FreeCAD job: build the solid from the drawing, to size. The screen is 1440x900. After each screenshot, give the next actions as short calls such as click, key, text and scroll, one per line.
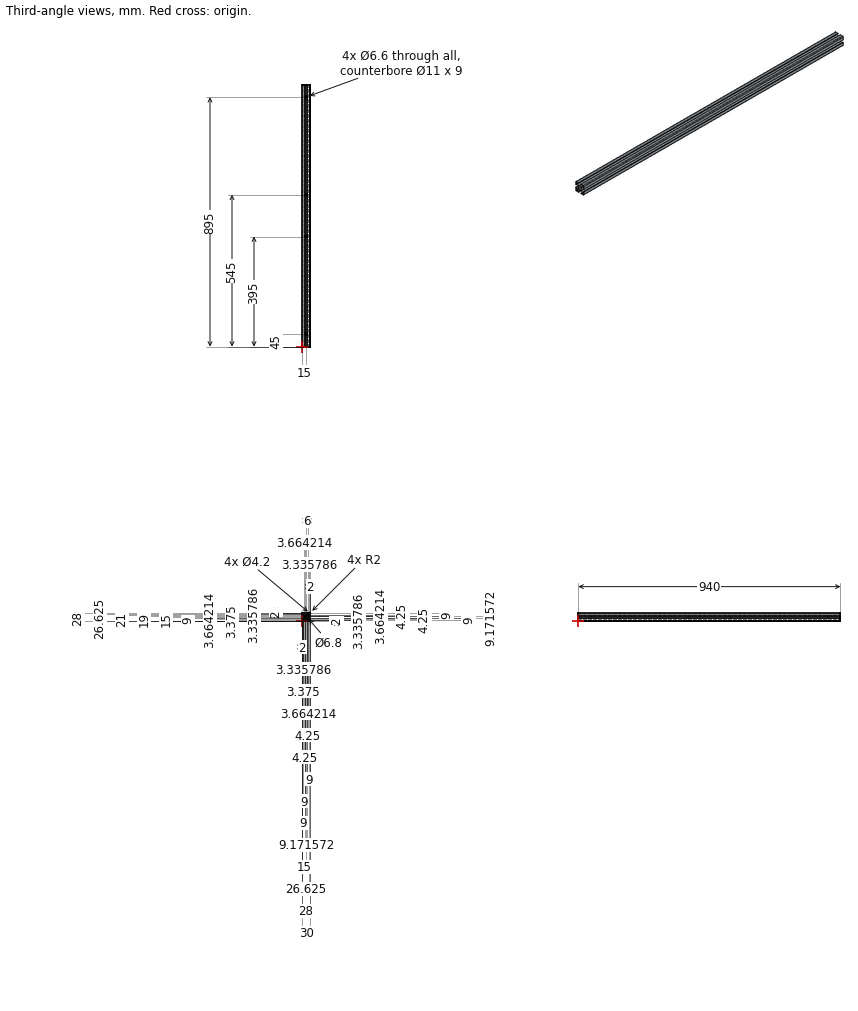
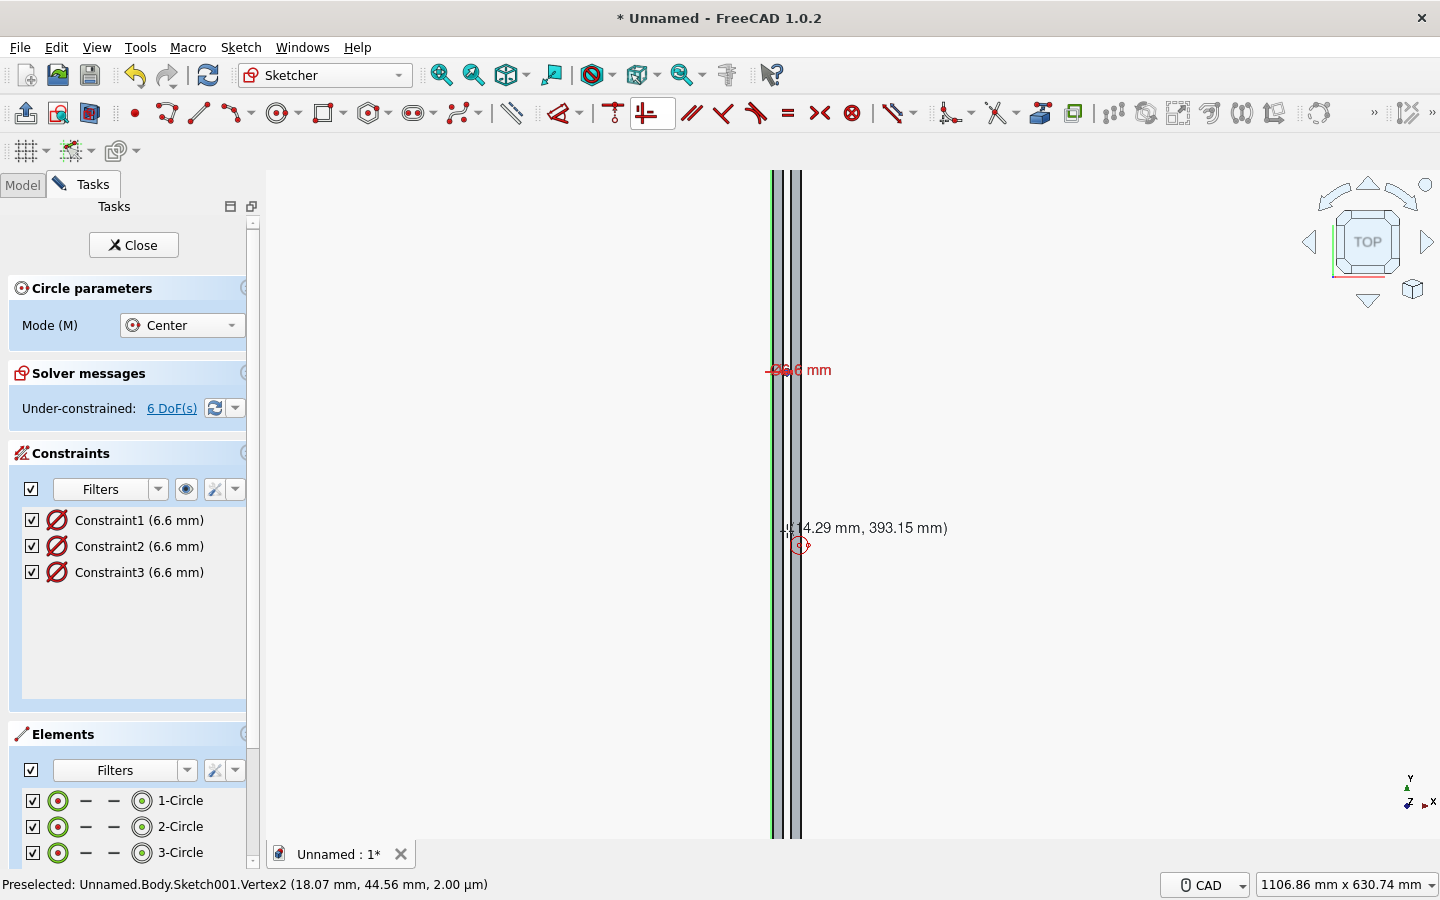
click(787, 531)
move(790, 528)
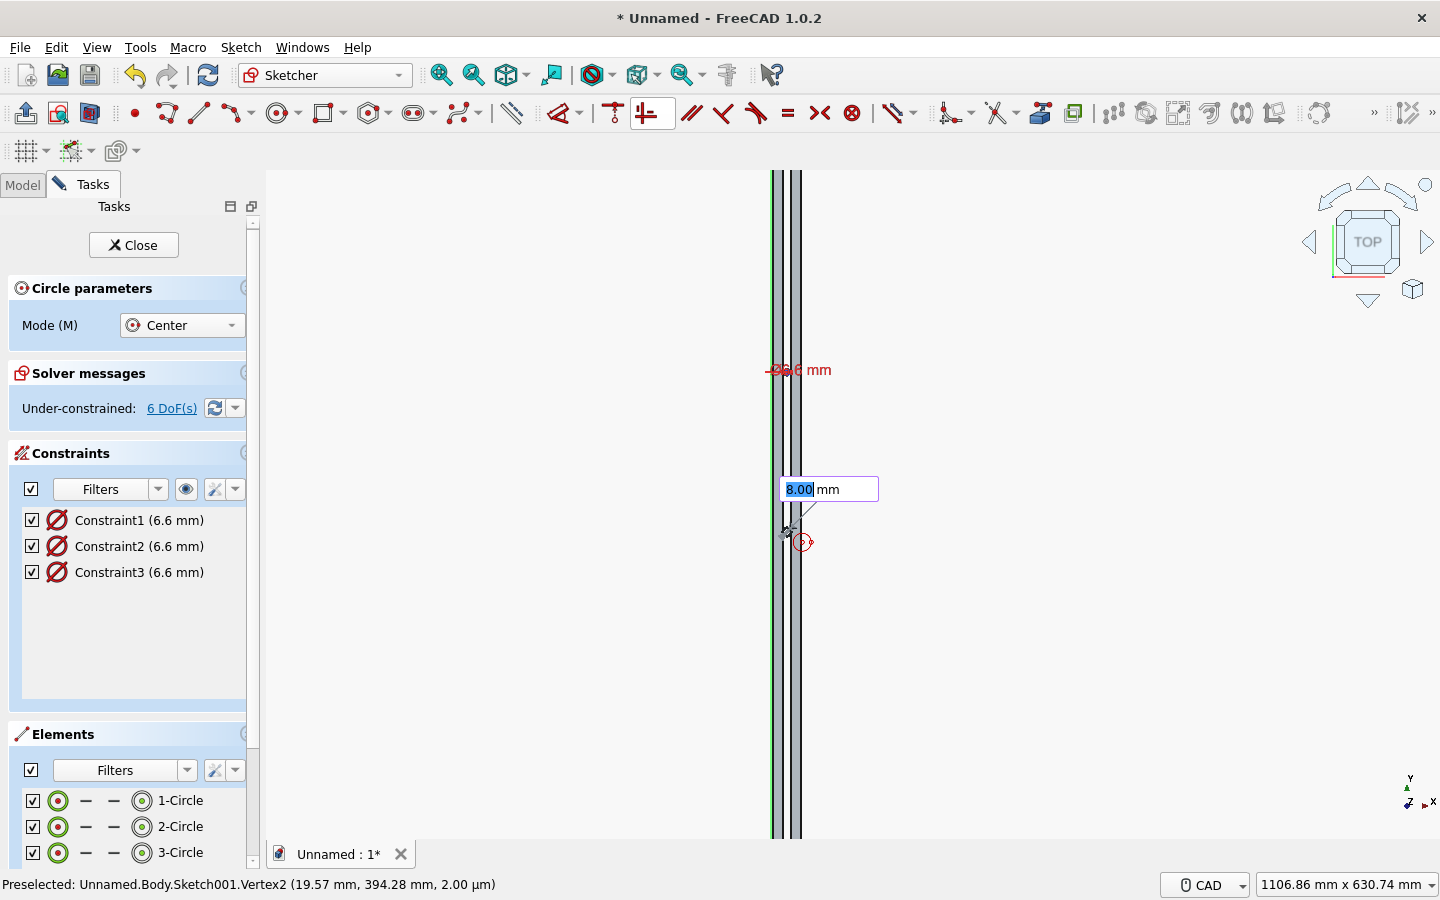
text(6.6)
key(Return)
key(Escape)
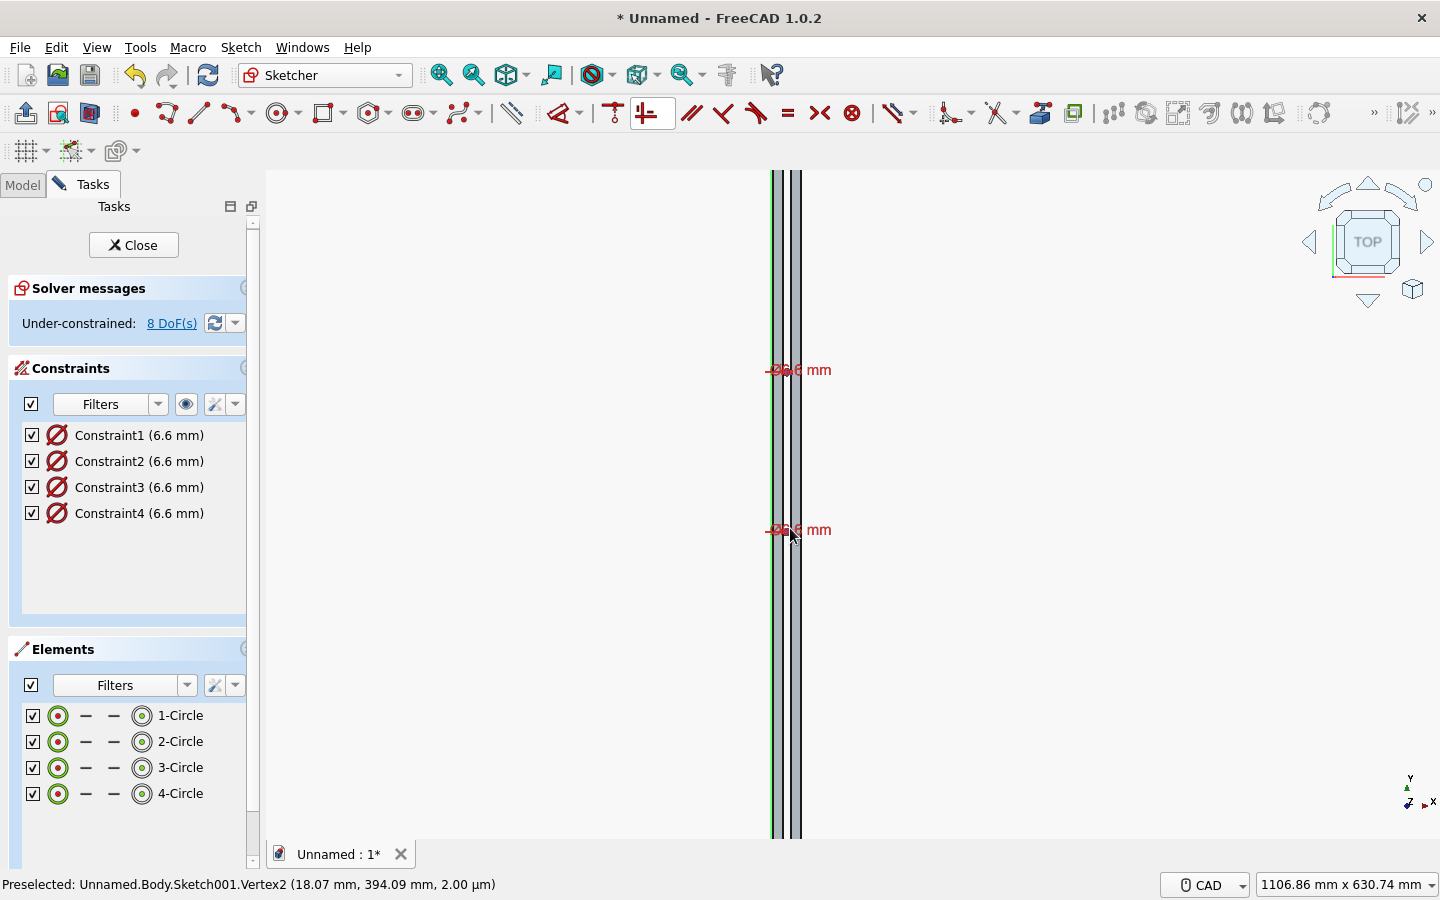
click(558, 114)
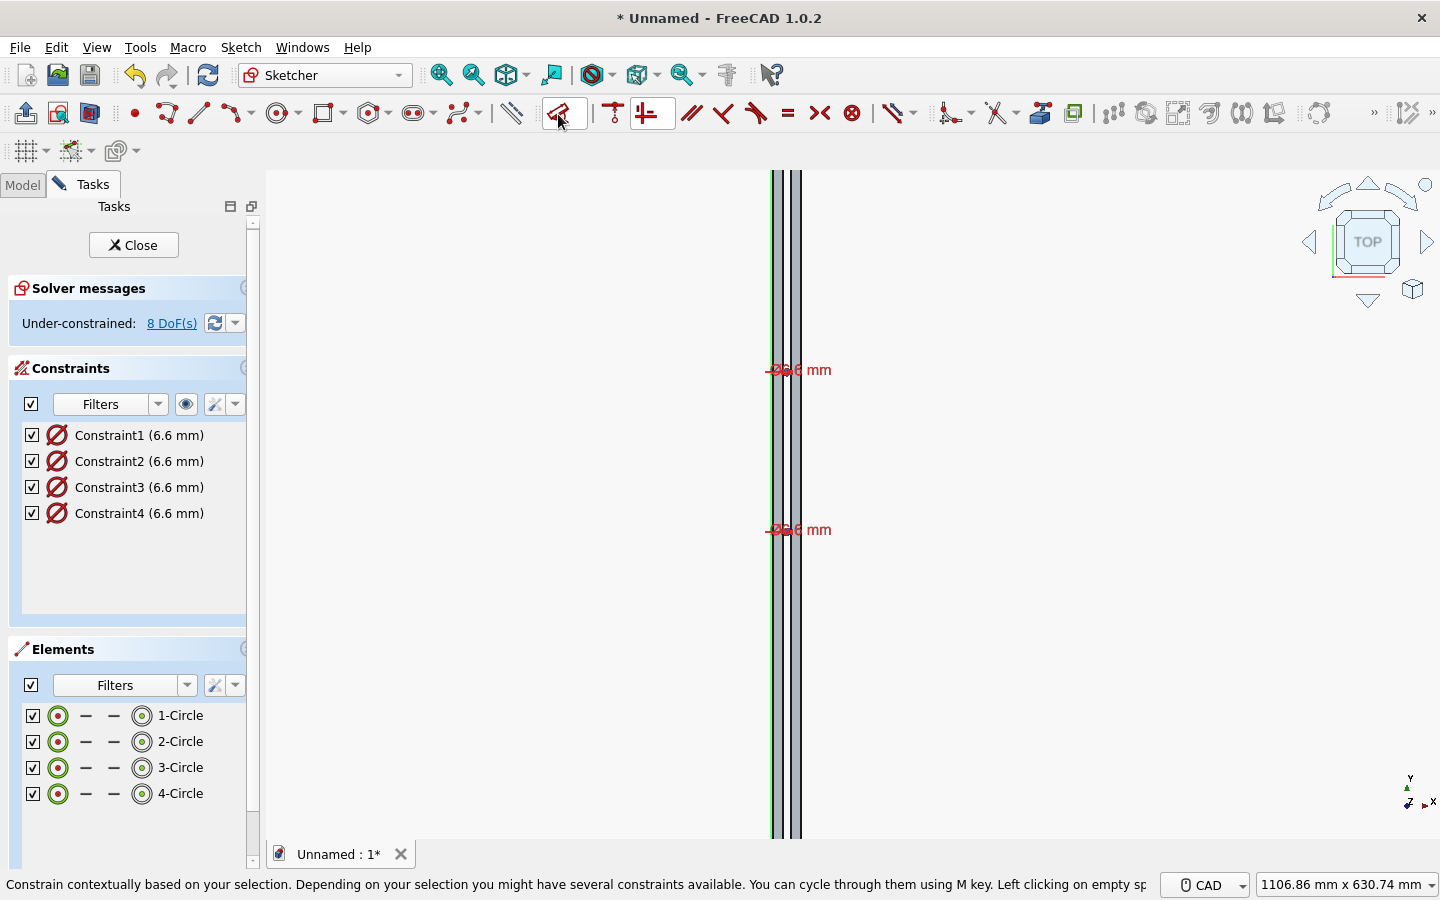
scroll(787, 530, down, 4)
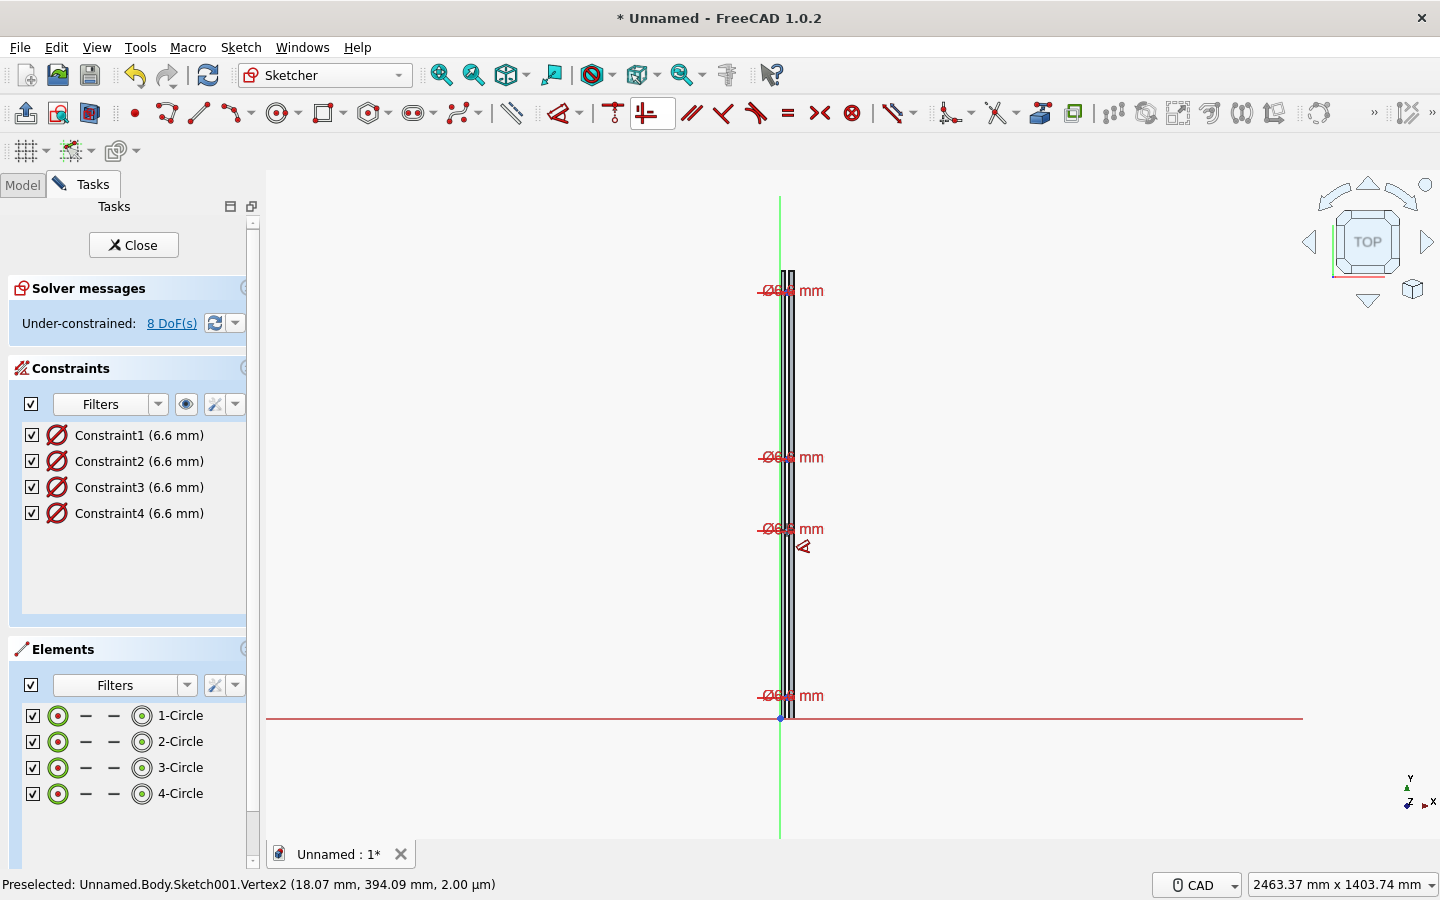
scroll(787, 293, up, 9)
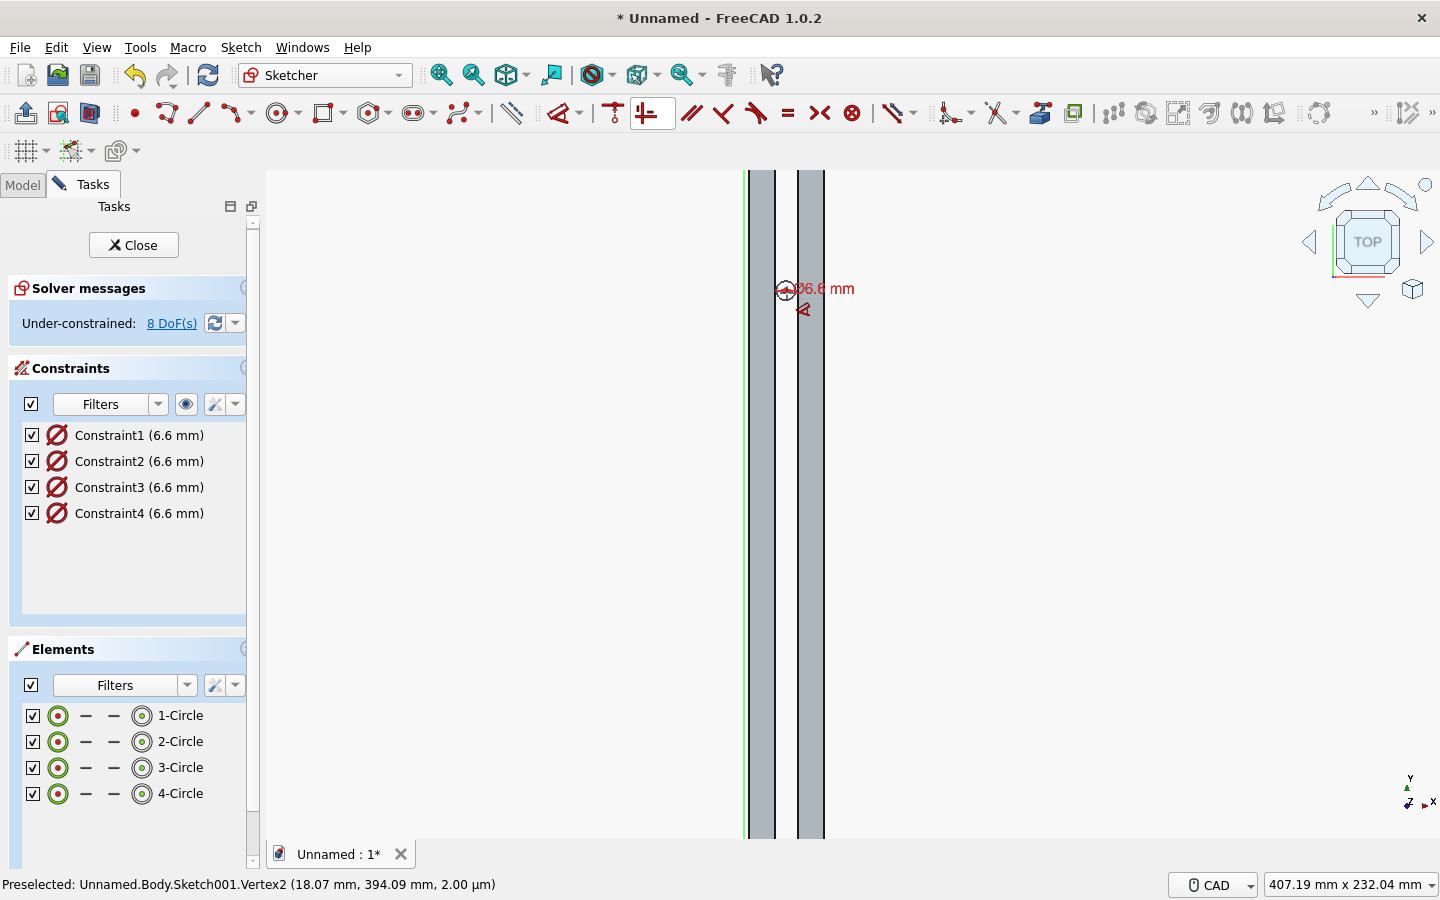
click(786, 291)
click(765, 257)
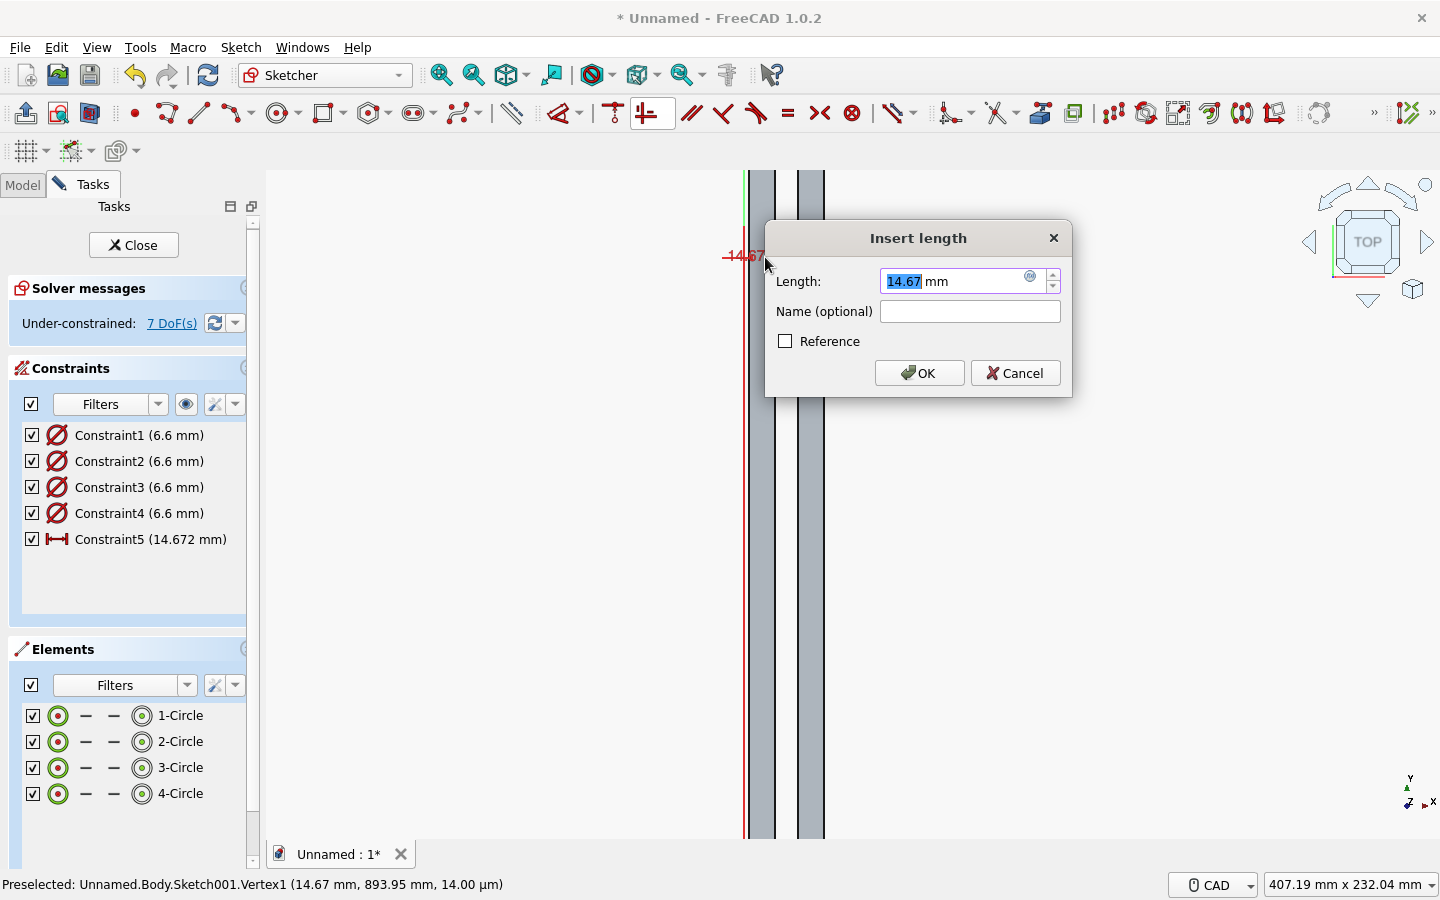
text(15)
key(Return)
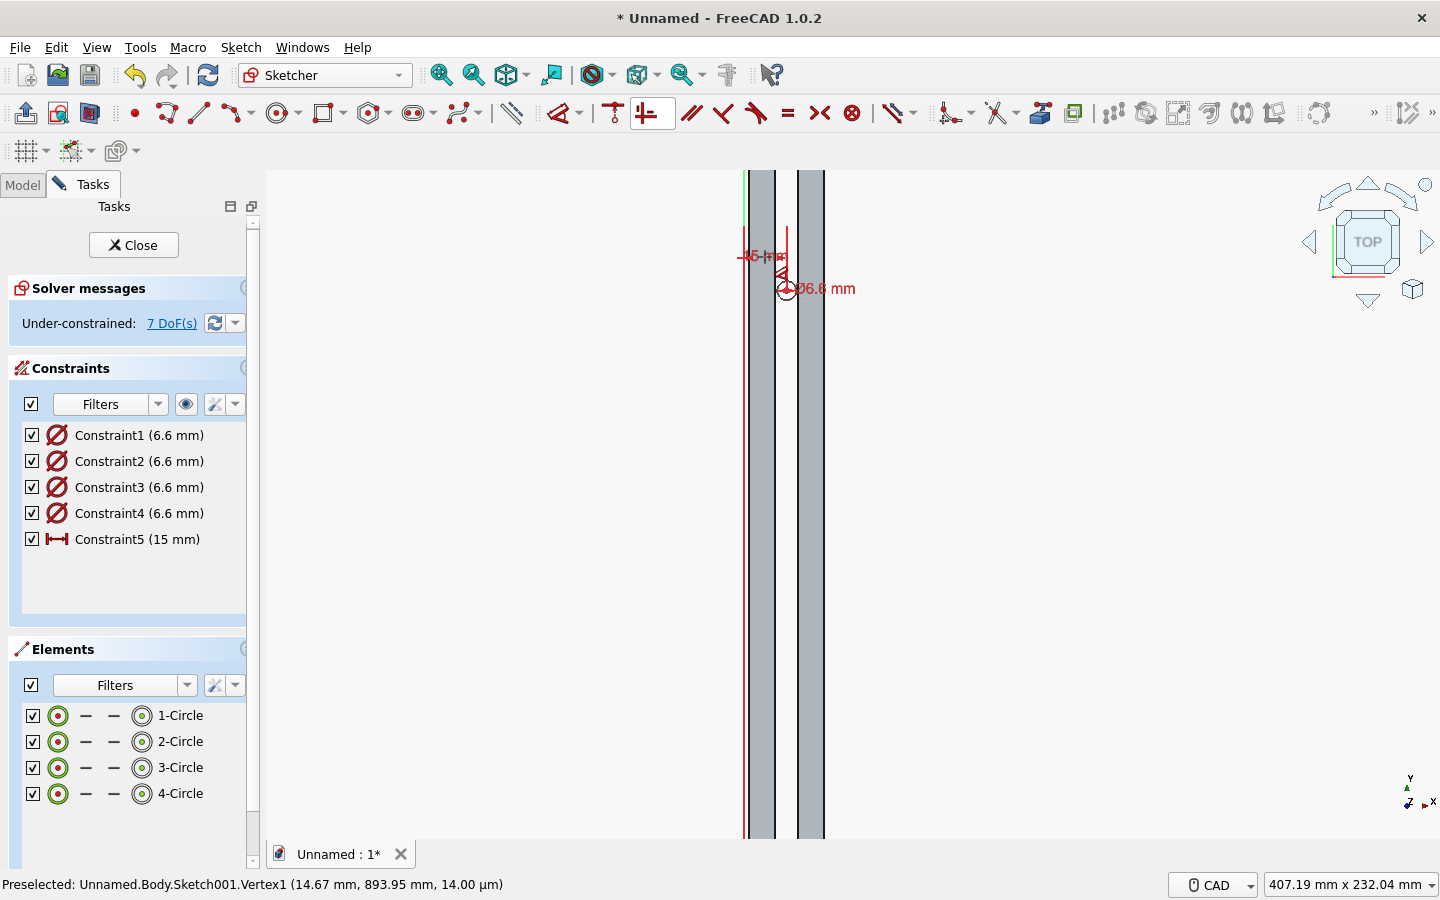
scroll(787, 293, down, 9)